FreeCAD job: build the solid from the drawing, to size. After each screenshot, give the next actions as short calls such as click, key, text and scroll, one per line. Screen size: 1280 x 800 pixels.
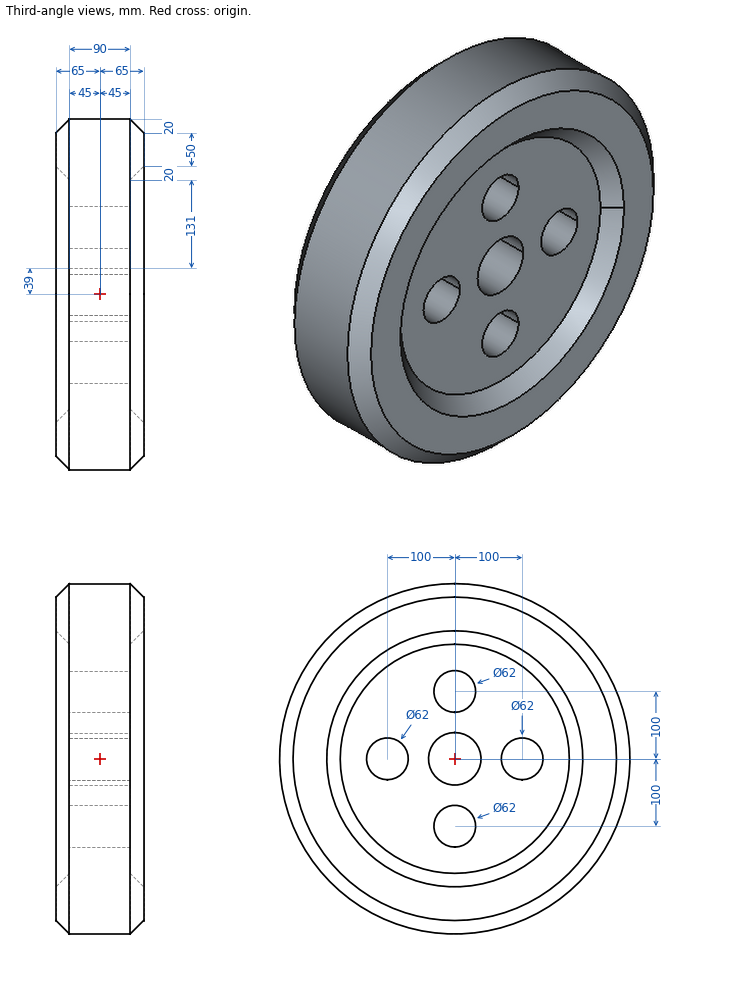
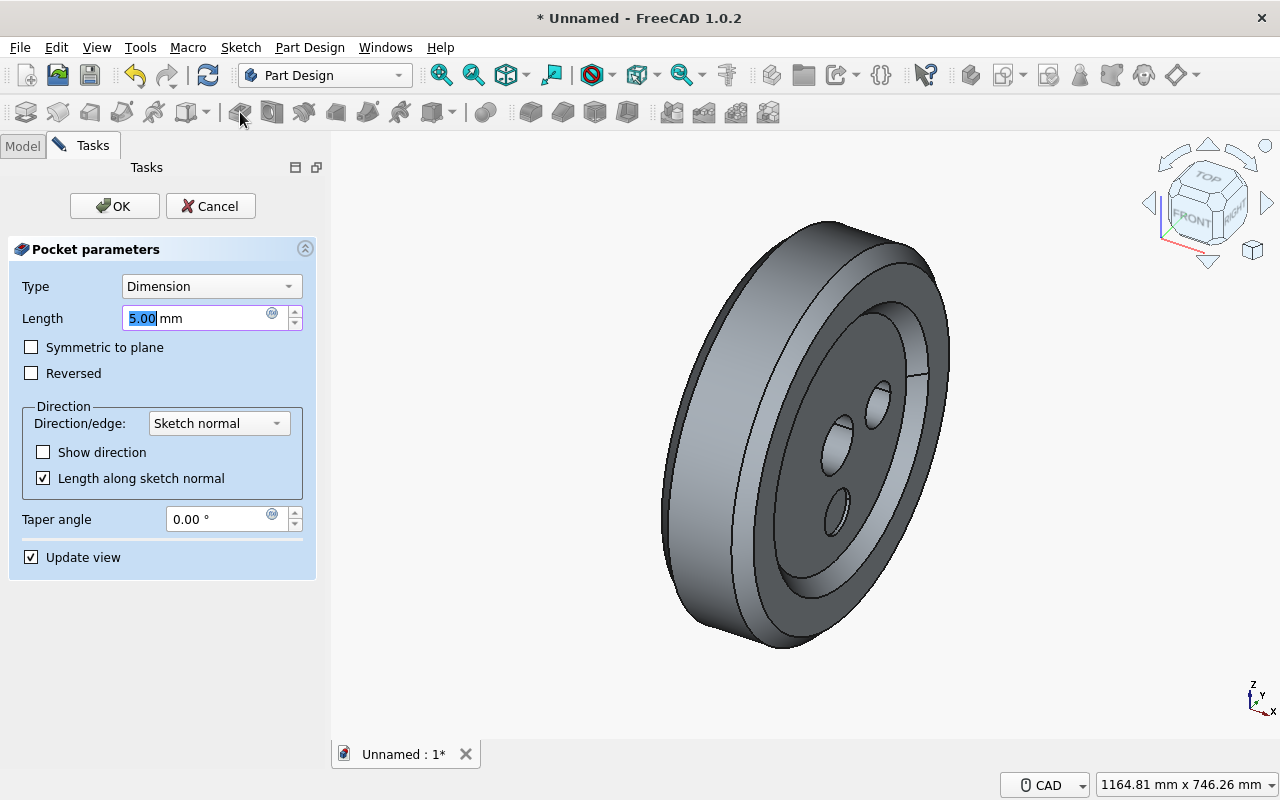
click(212, 286)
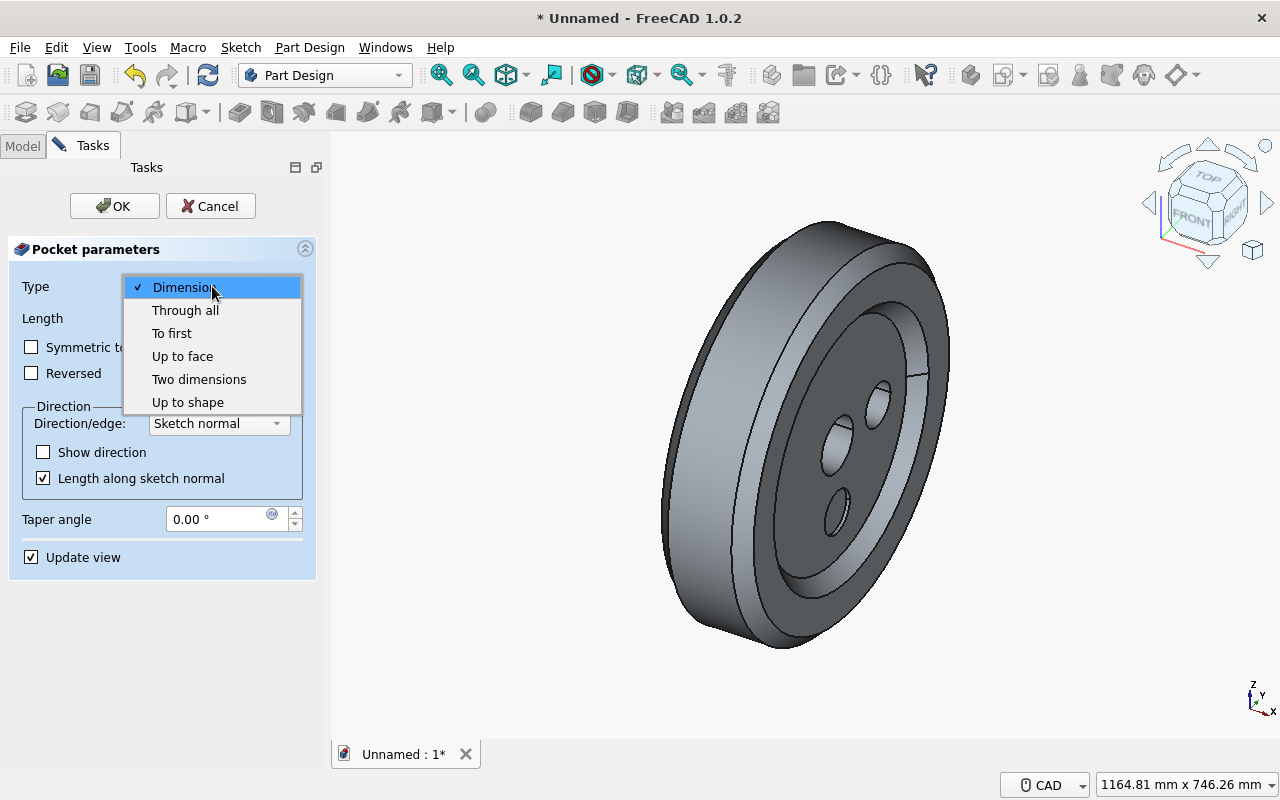
click(212, 334)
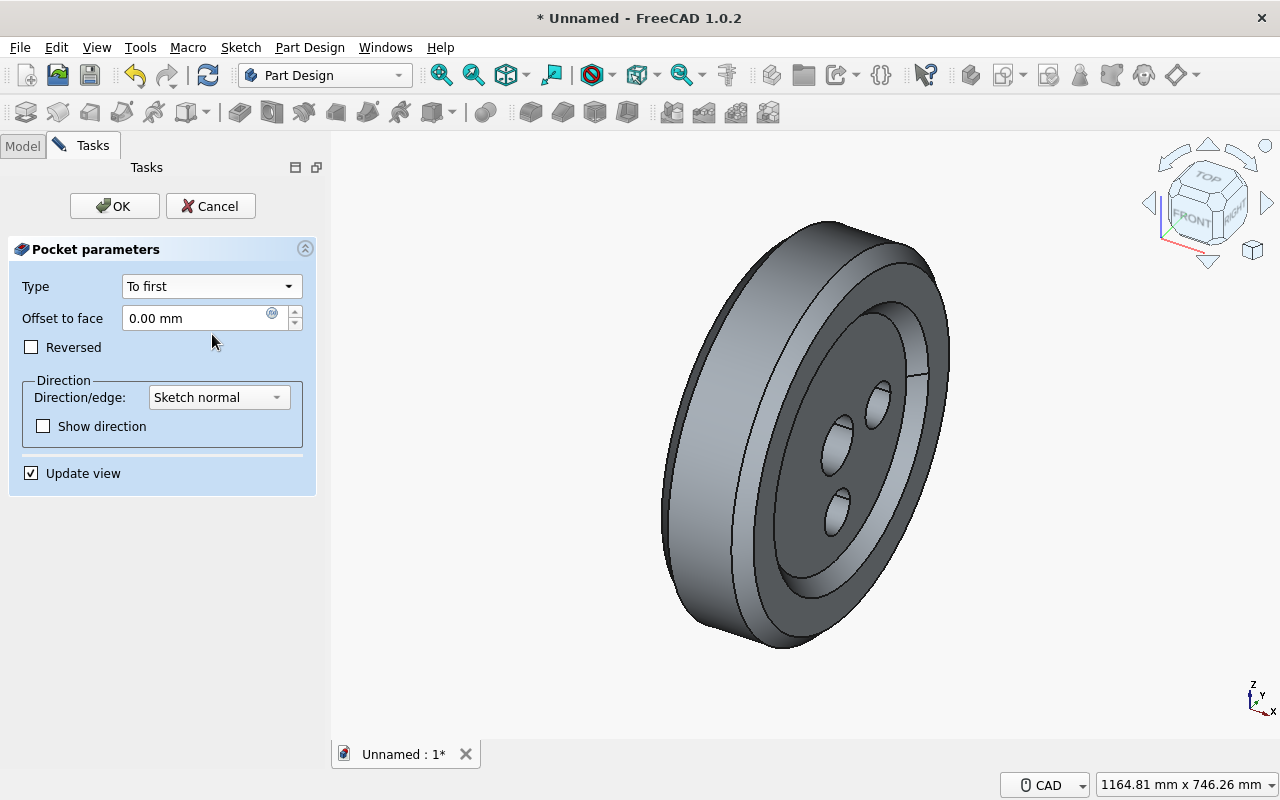
click(115, 206)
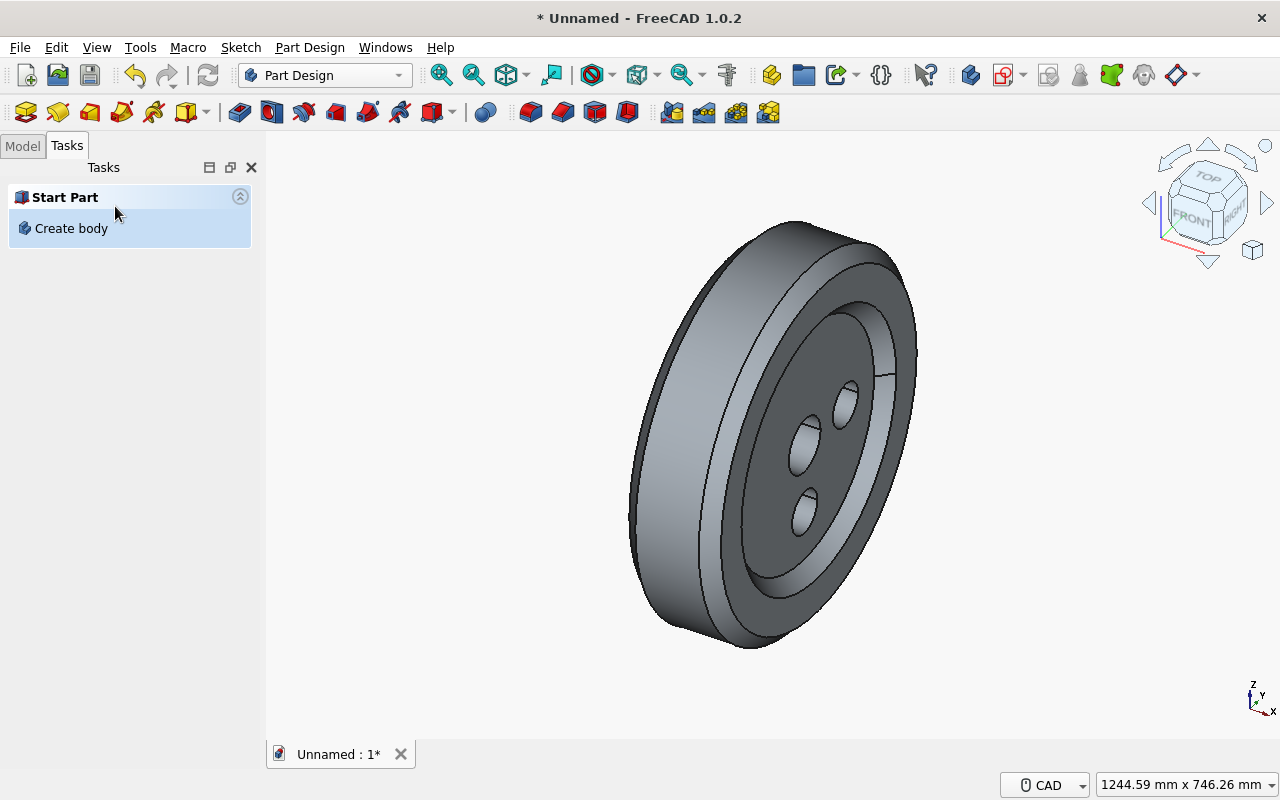
click(825, 360)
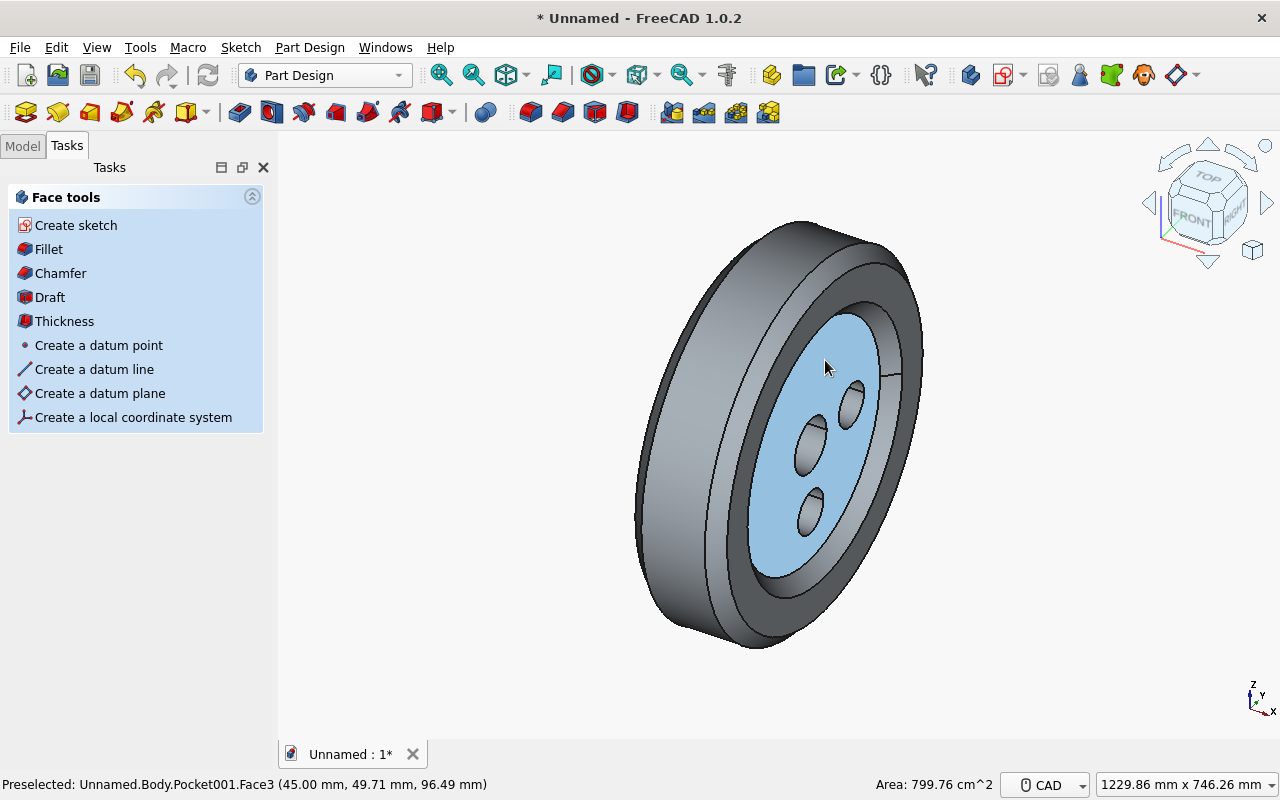
click(1004, 76)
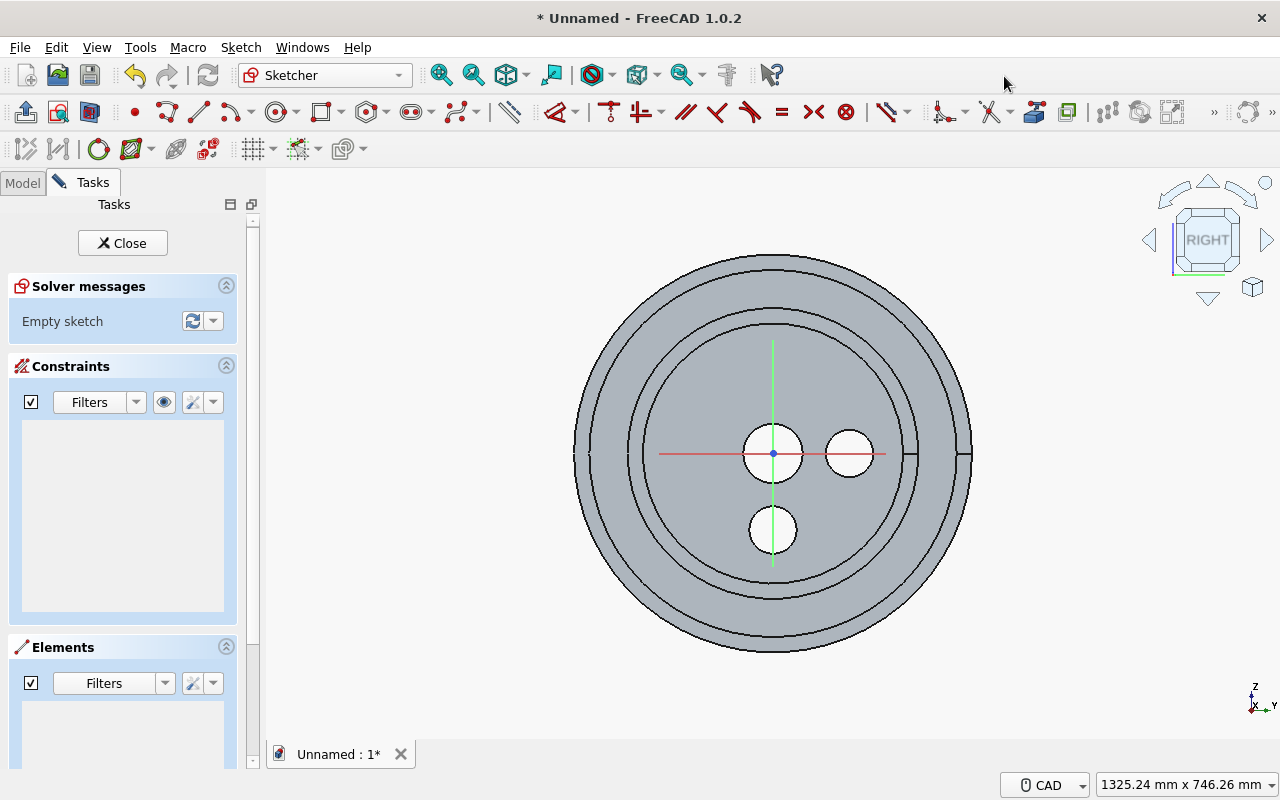
scroll(727, 454, up, 9)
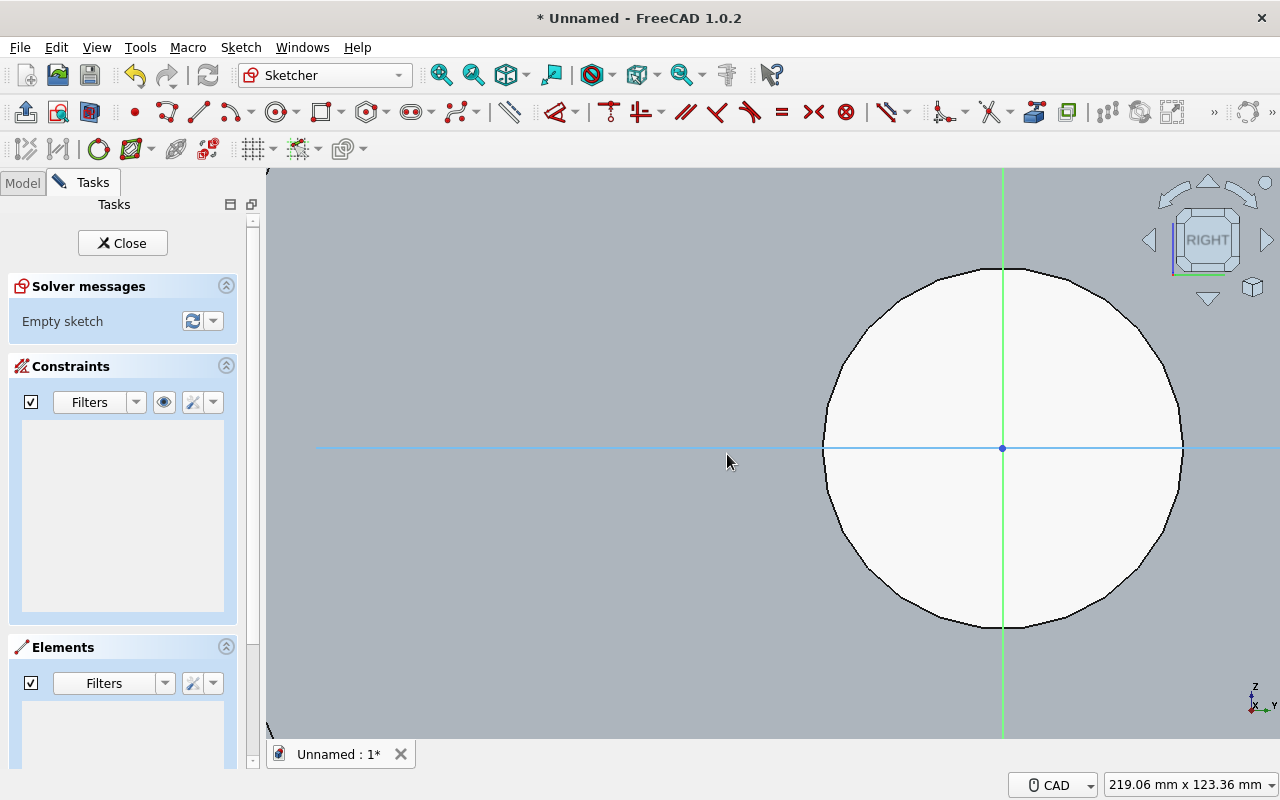
key(g)
key(c)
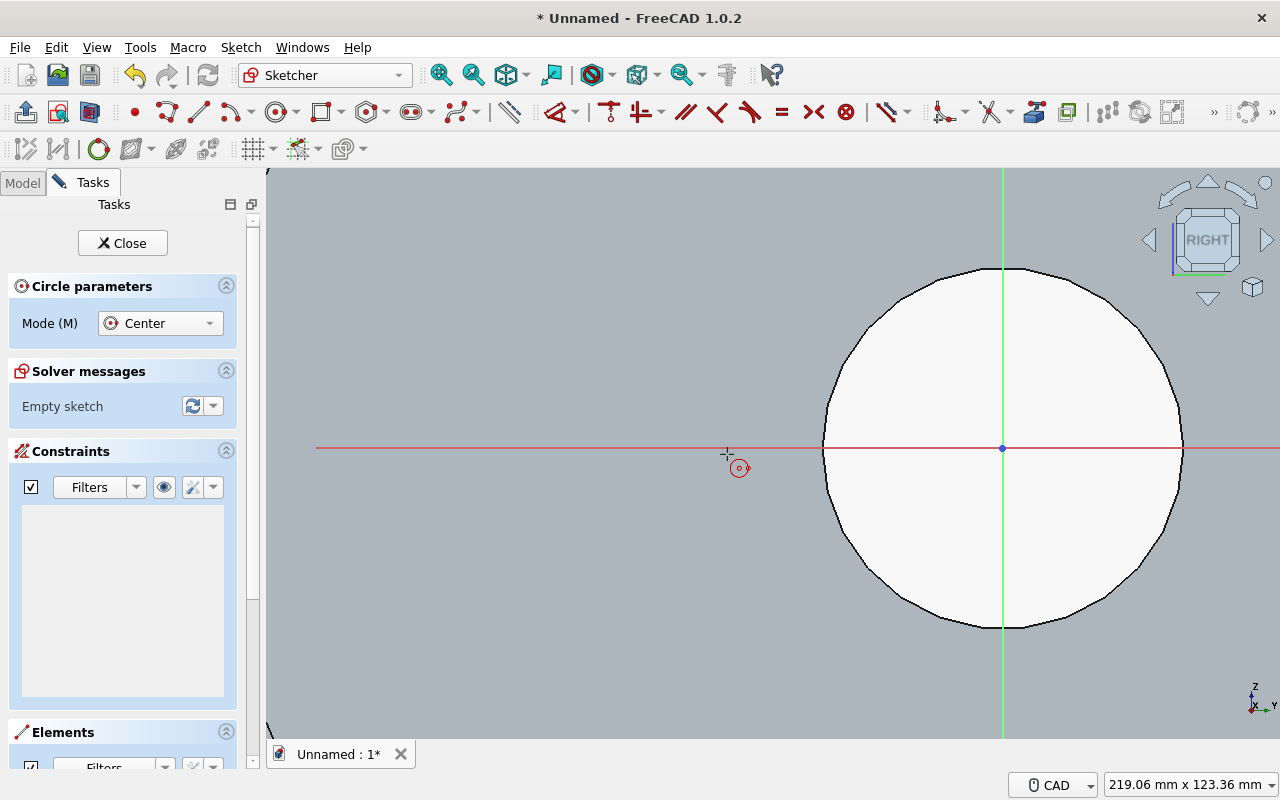
click(540, 448)
click(642, 347)
key(Escape)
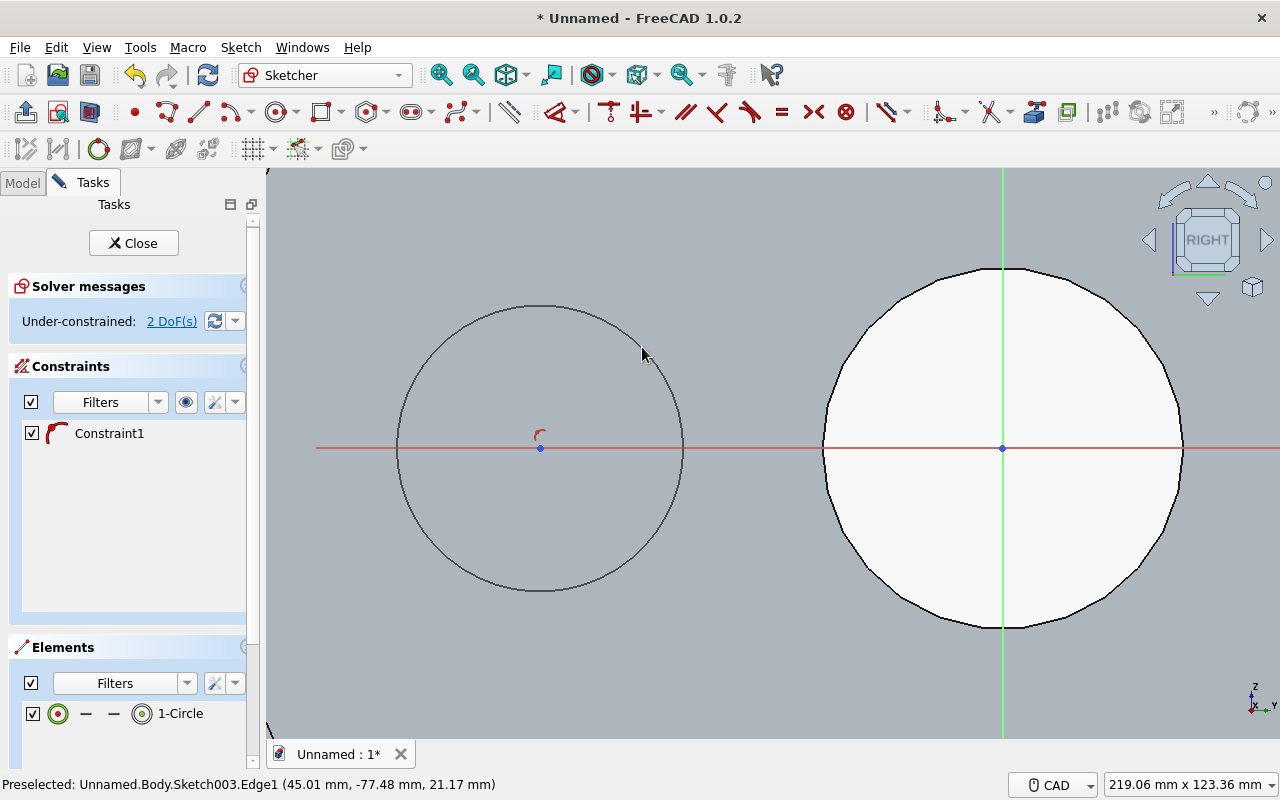
click(556, 112)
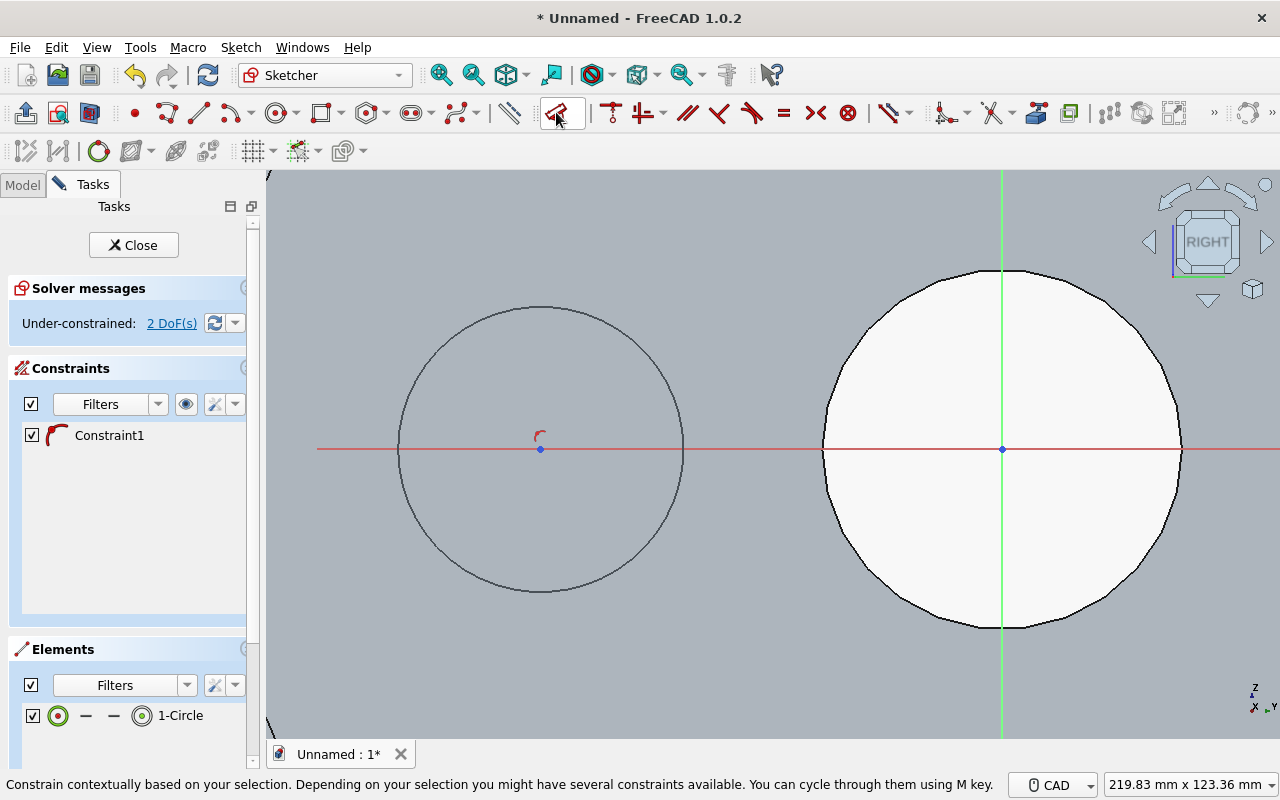
click(641, 348)
click(663, 325)